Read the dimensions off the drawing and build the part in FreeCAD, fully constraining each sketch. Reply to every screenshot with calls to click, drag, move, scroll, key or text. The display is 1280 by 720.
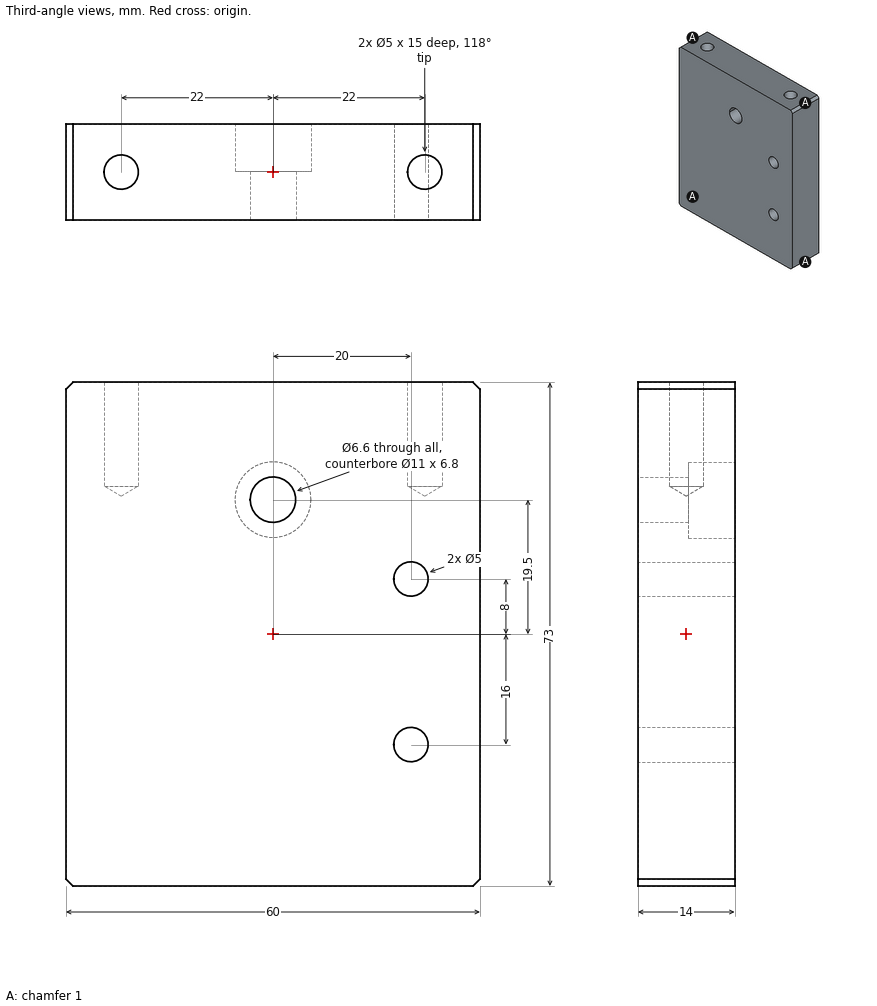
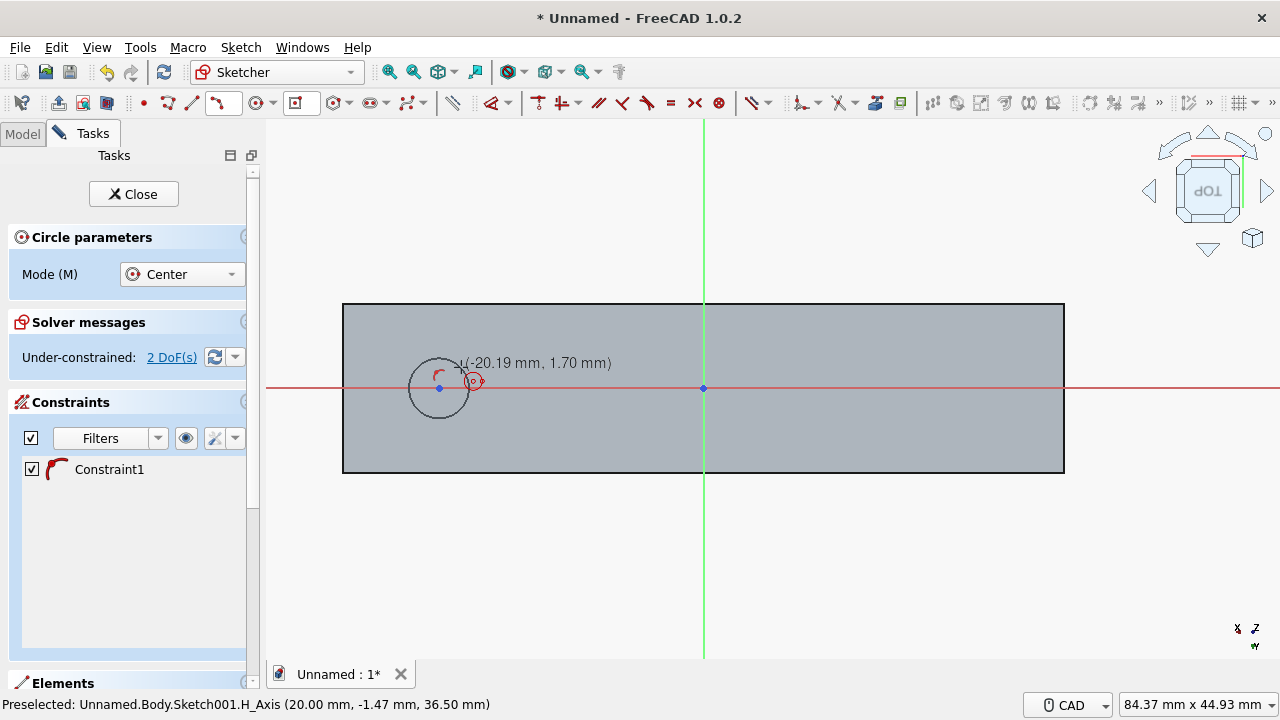
click(968, 388)
click(989, 367)
key(Escape)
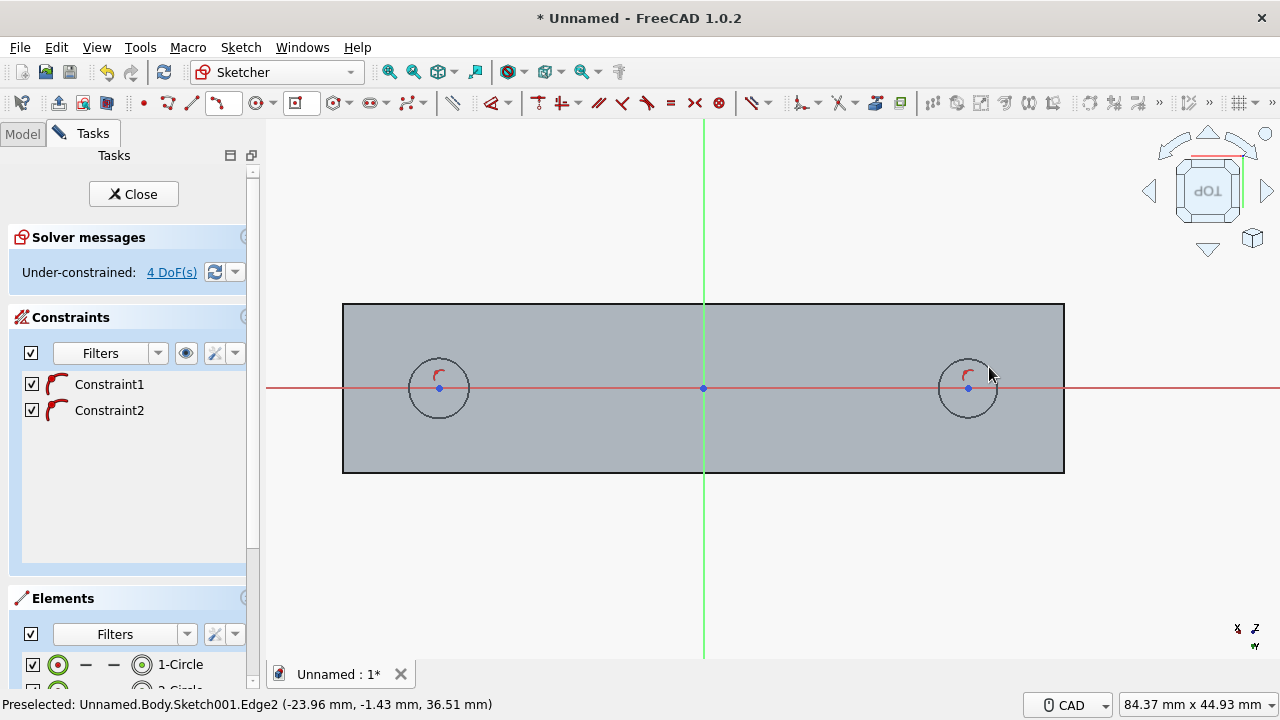
click(460, 367)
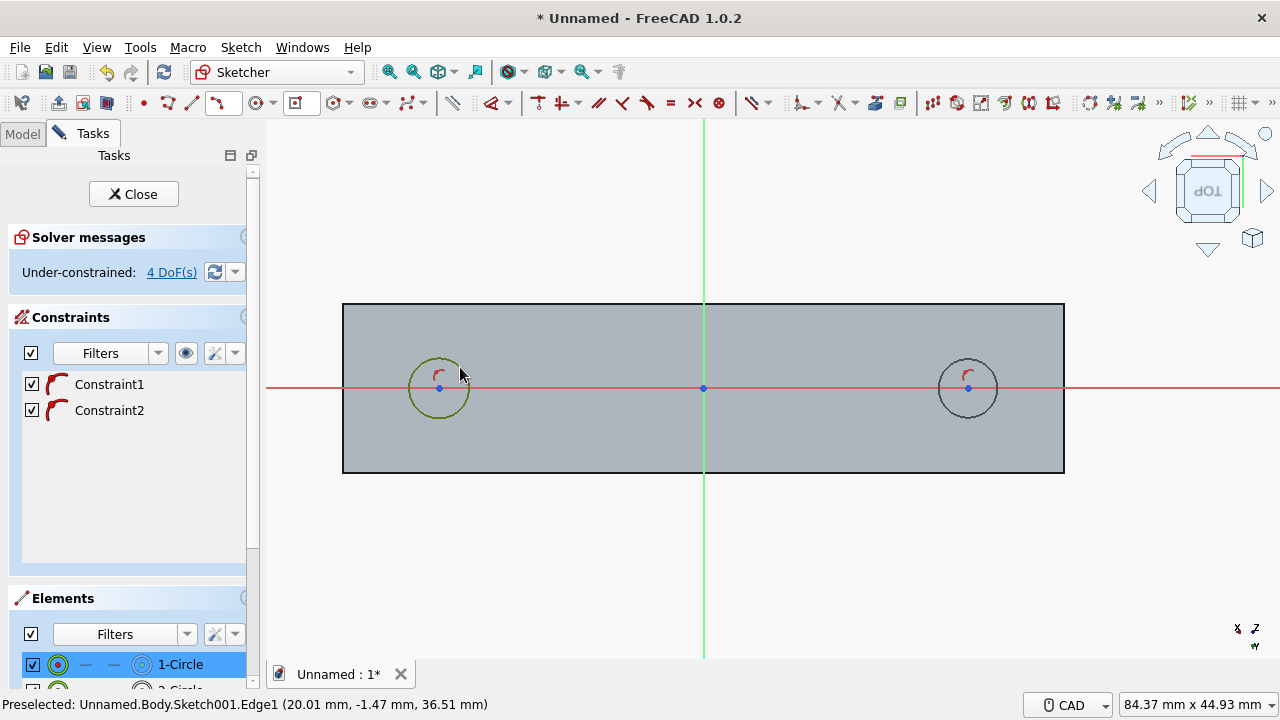
click(989, 368)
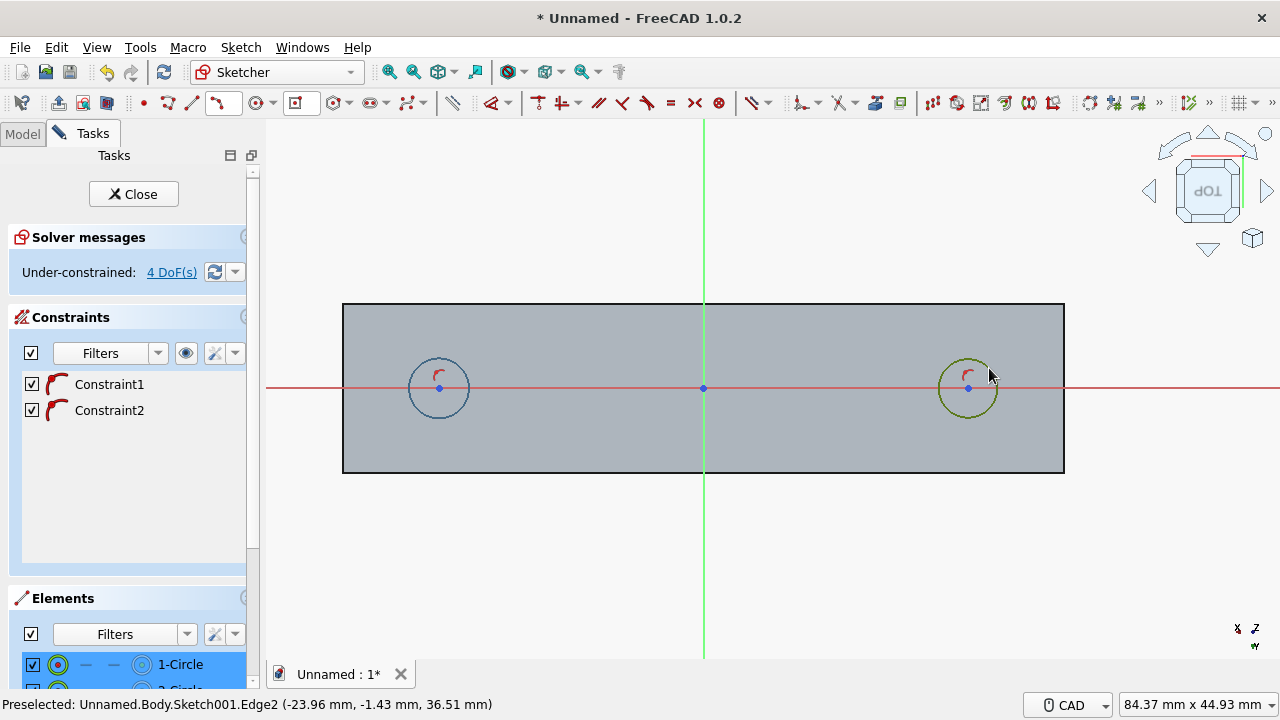
click(672, 104)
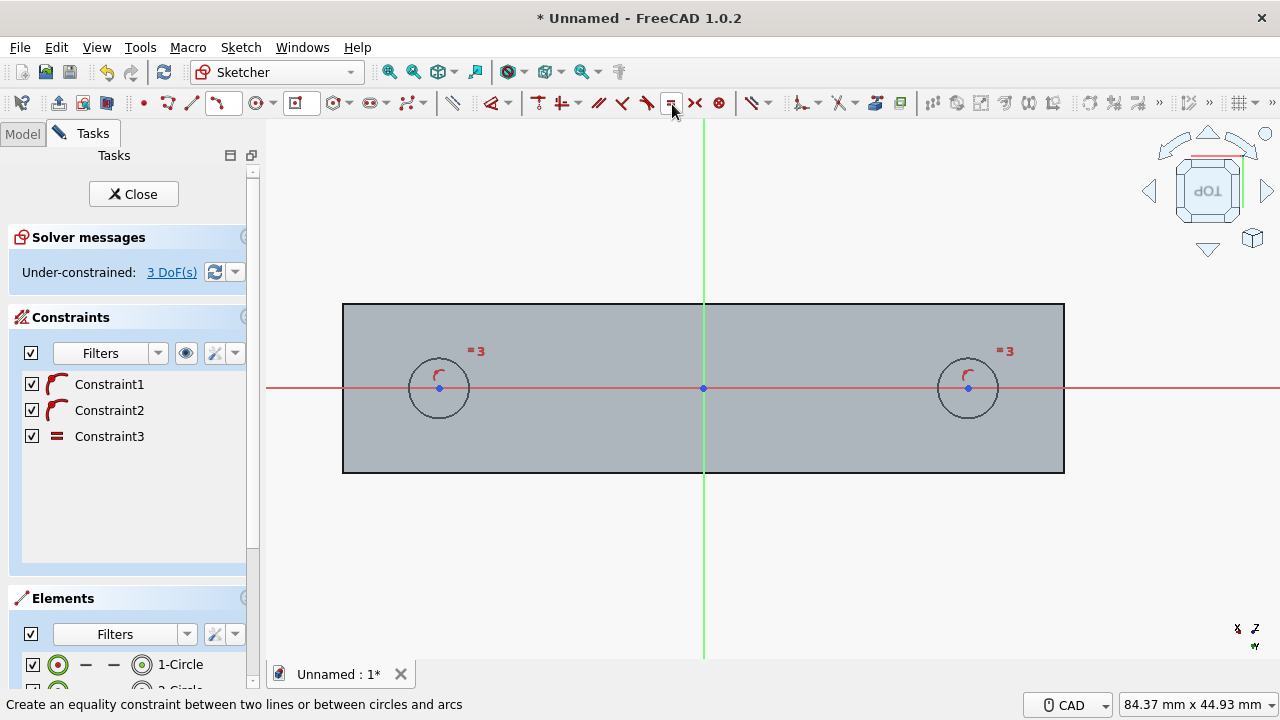
click(492, 104)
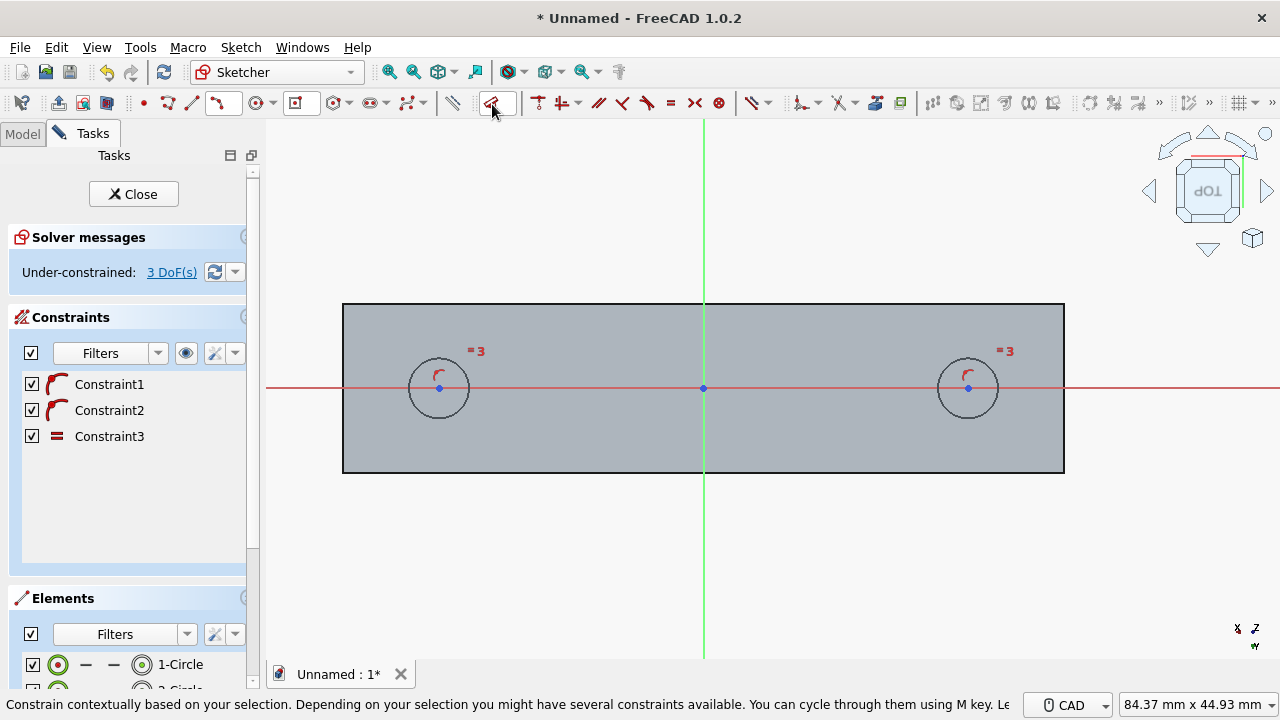
click(460, 367)
click(482, 344)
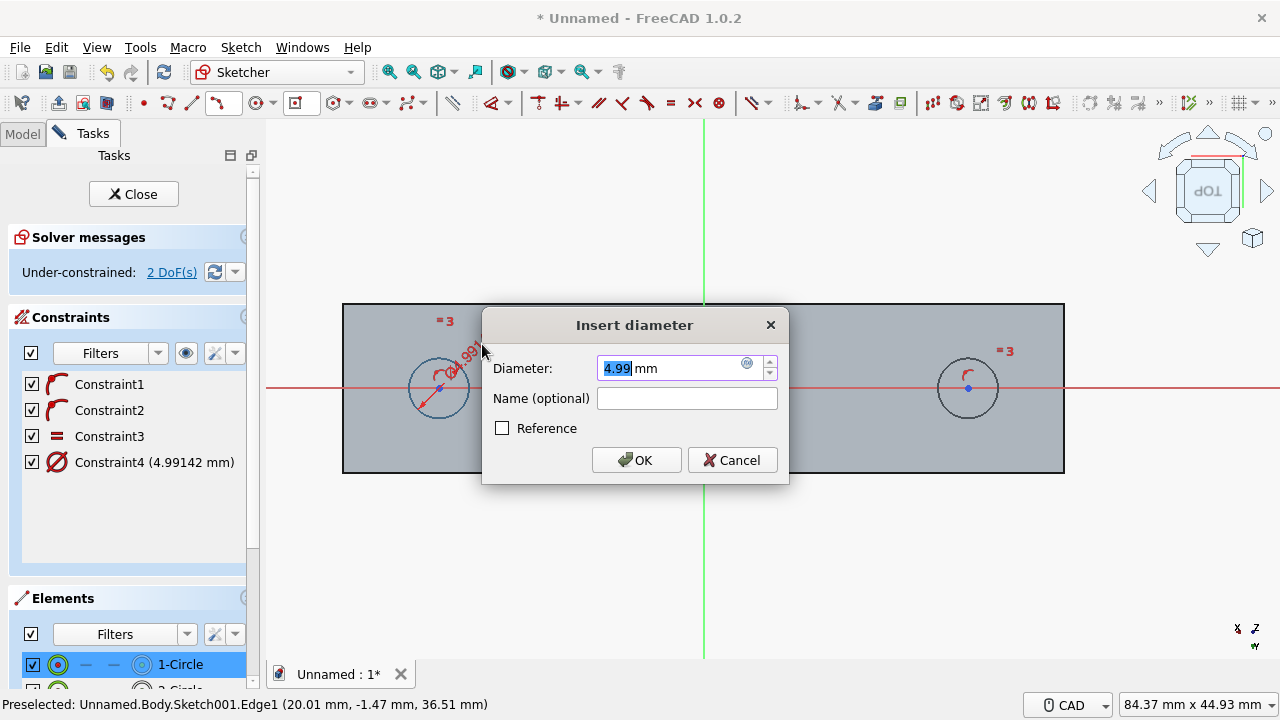
text(5)
key(Return)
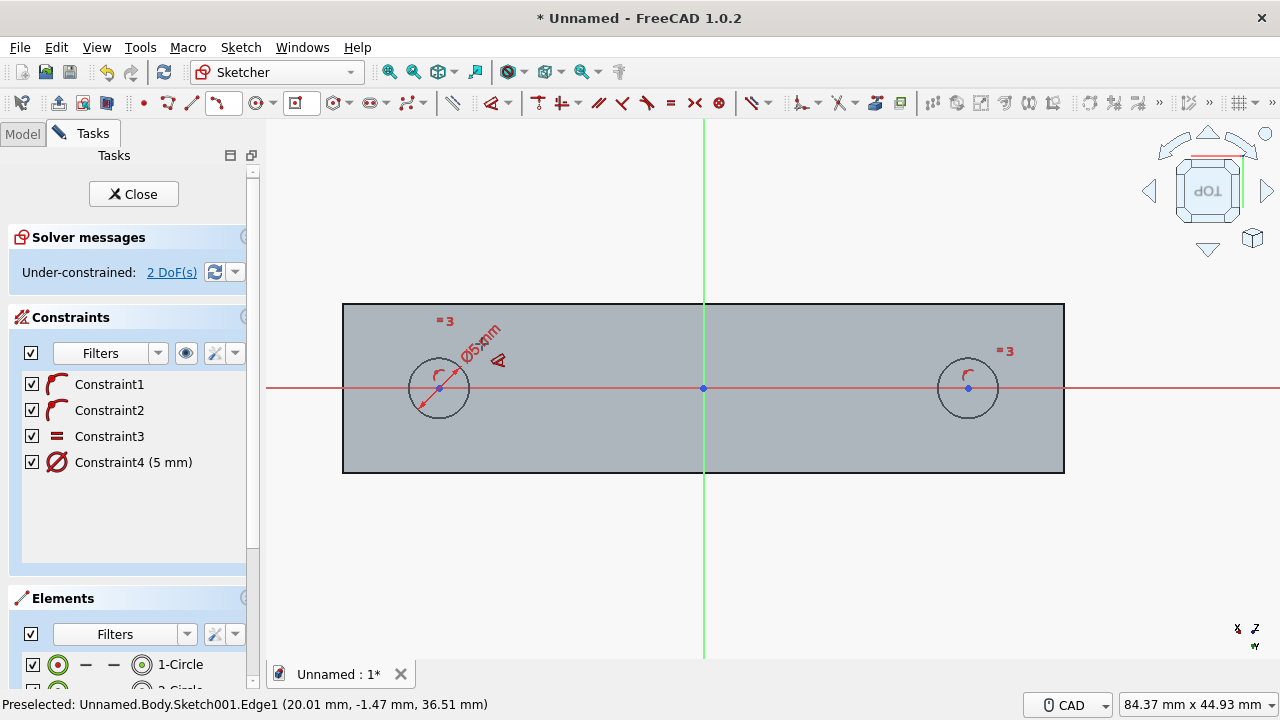
click(439, 388)
click(571, 422)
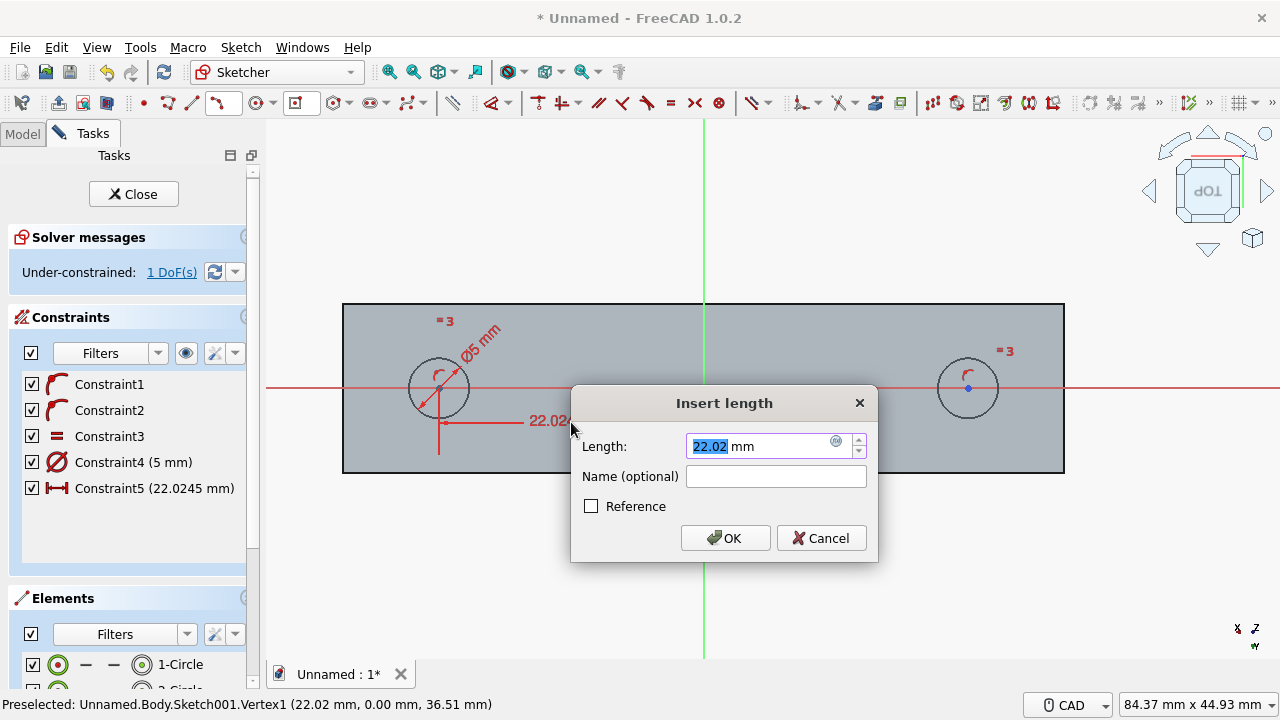
text(22)
key(Return)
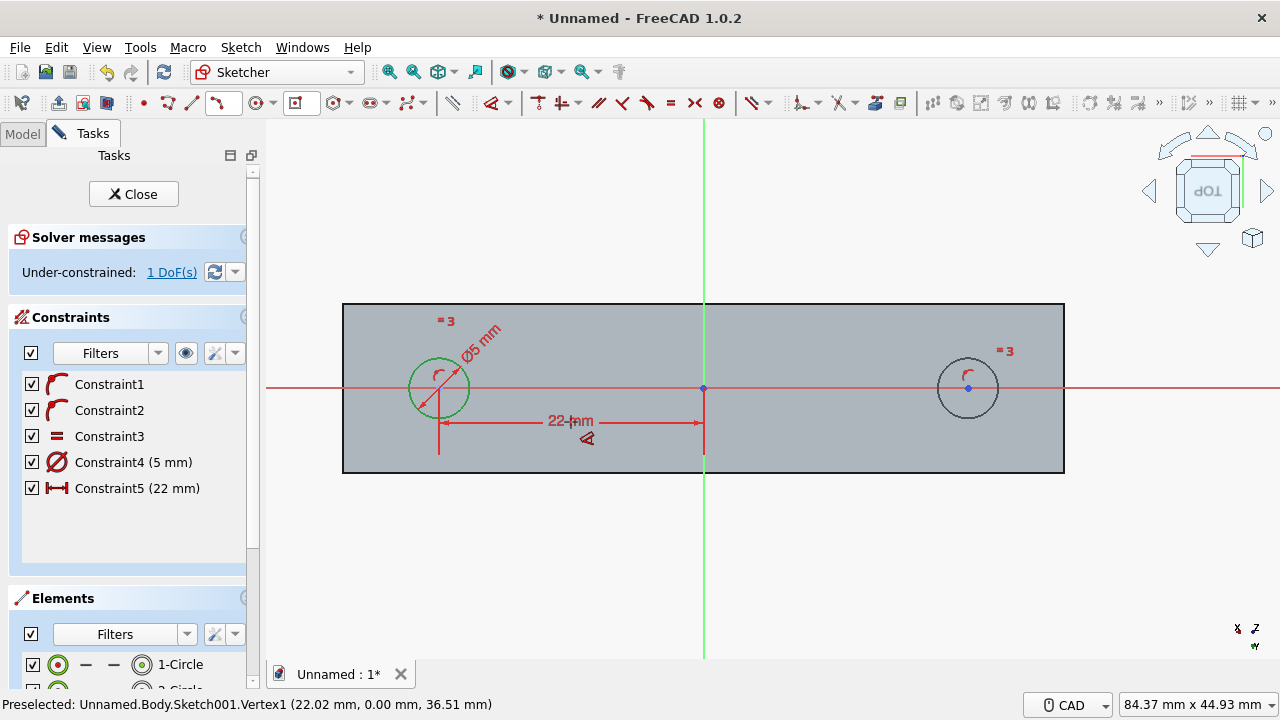
click(968, 388)
click(836, 422)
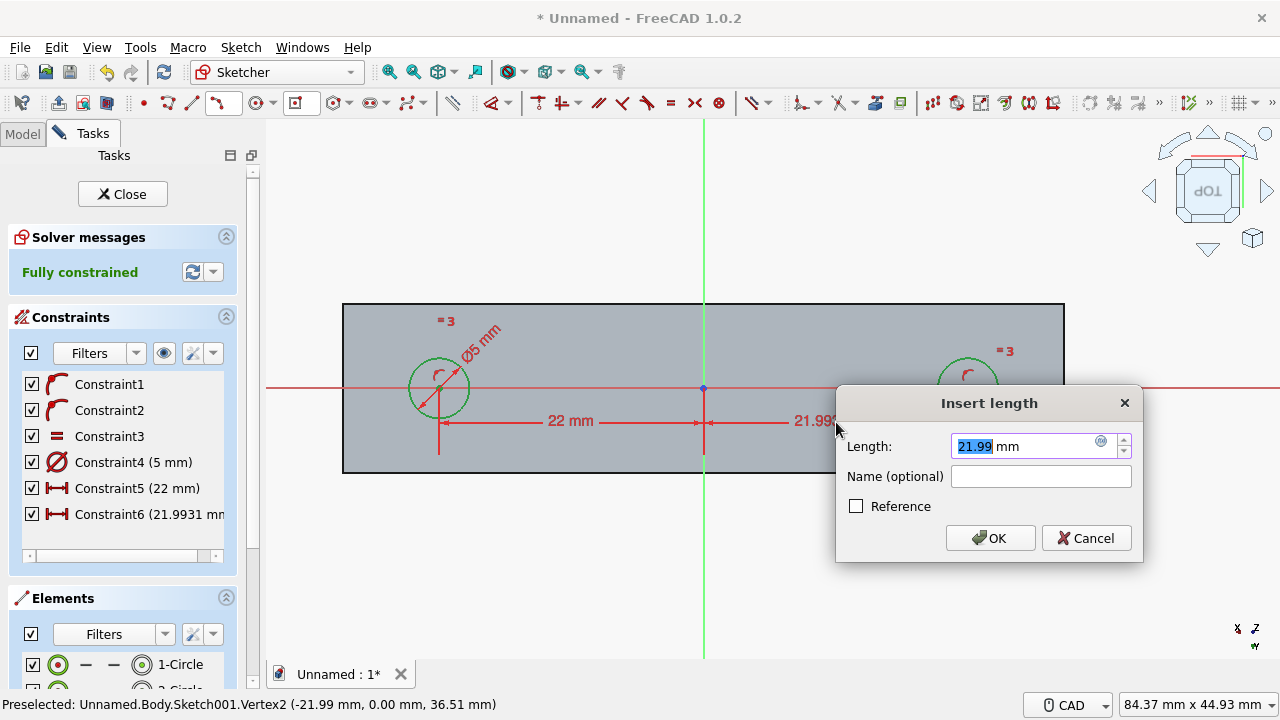
text(22)
key(Return)
key(Escape)